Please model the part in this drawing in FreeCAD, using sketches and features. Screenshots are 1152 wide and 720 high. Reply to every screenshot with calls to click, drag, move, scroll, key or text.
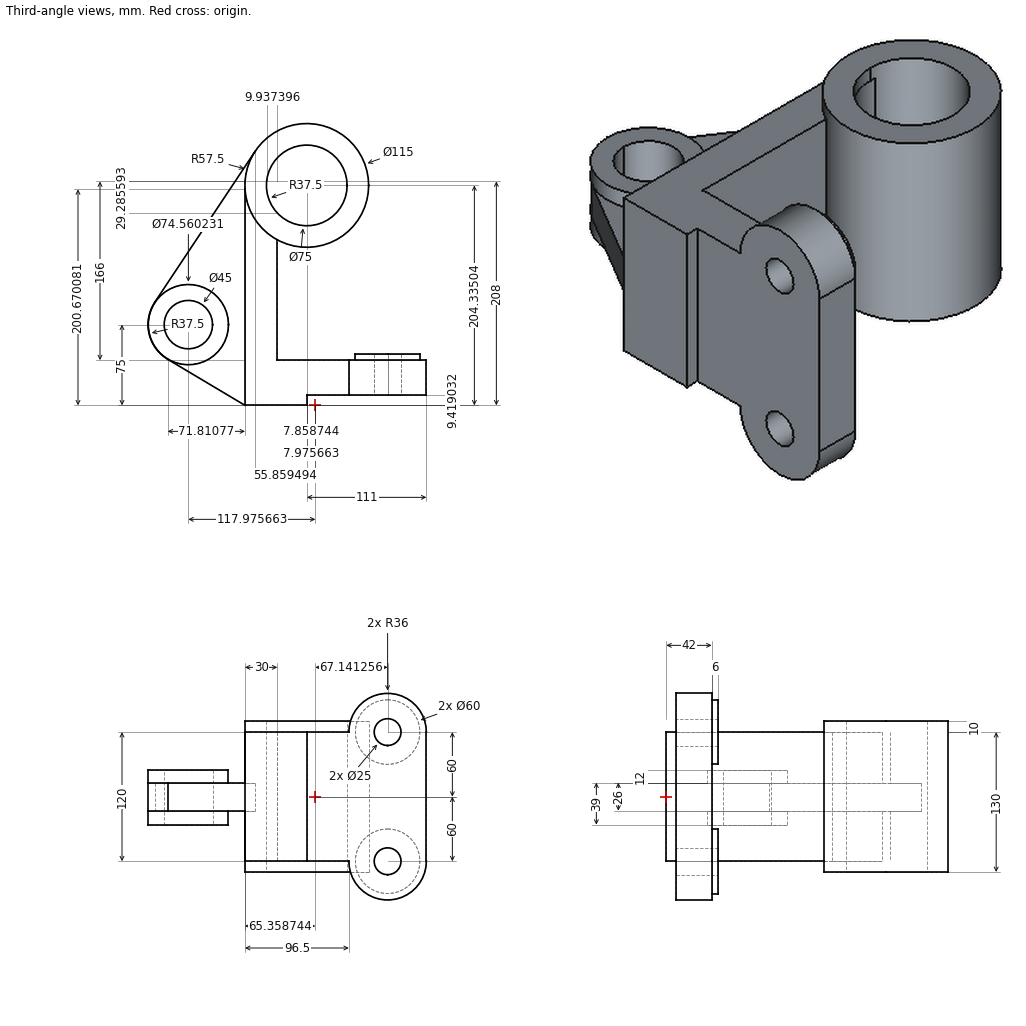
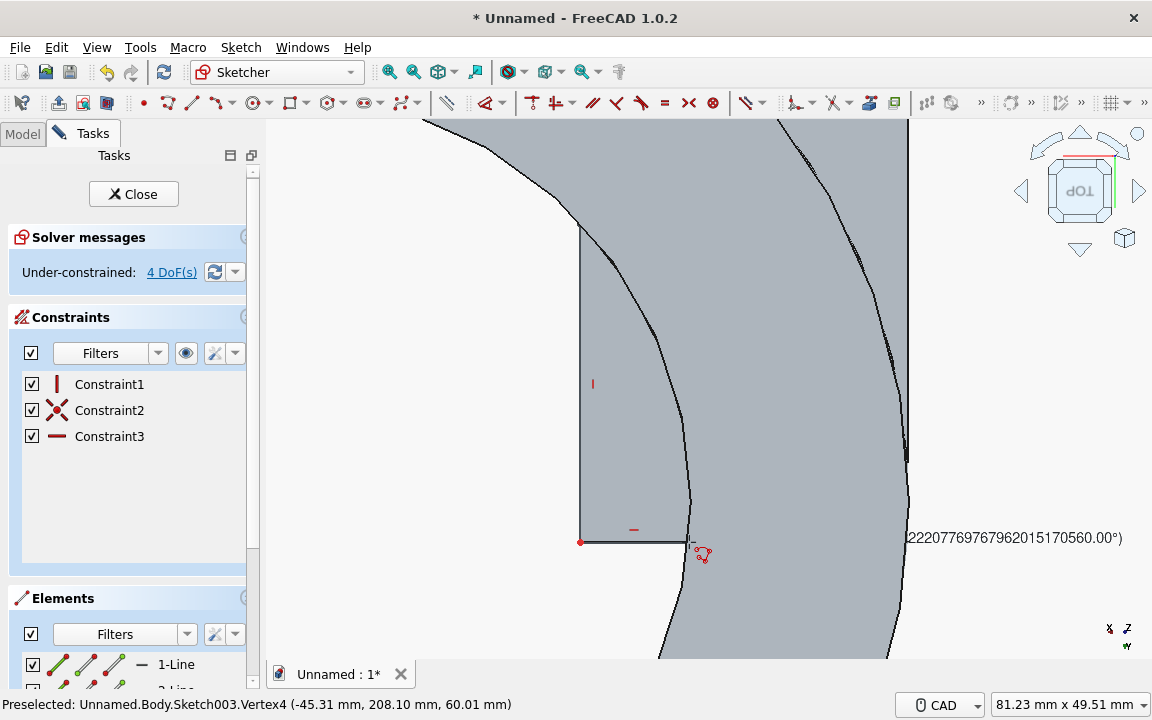
click(216, 104)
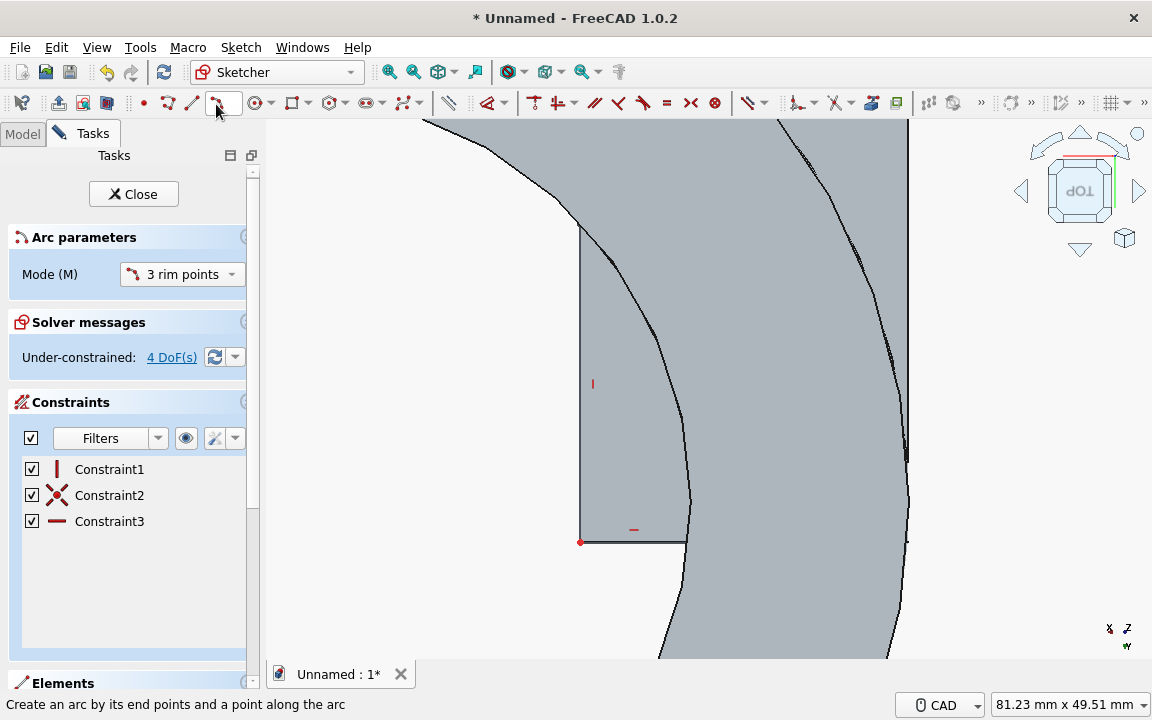
click(689, 543)
click(580, 224)
click(669, 371)
key(Escape)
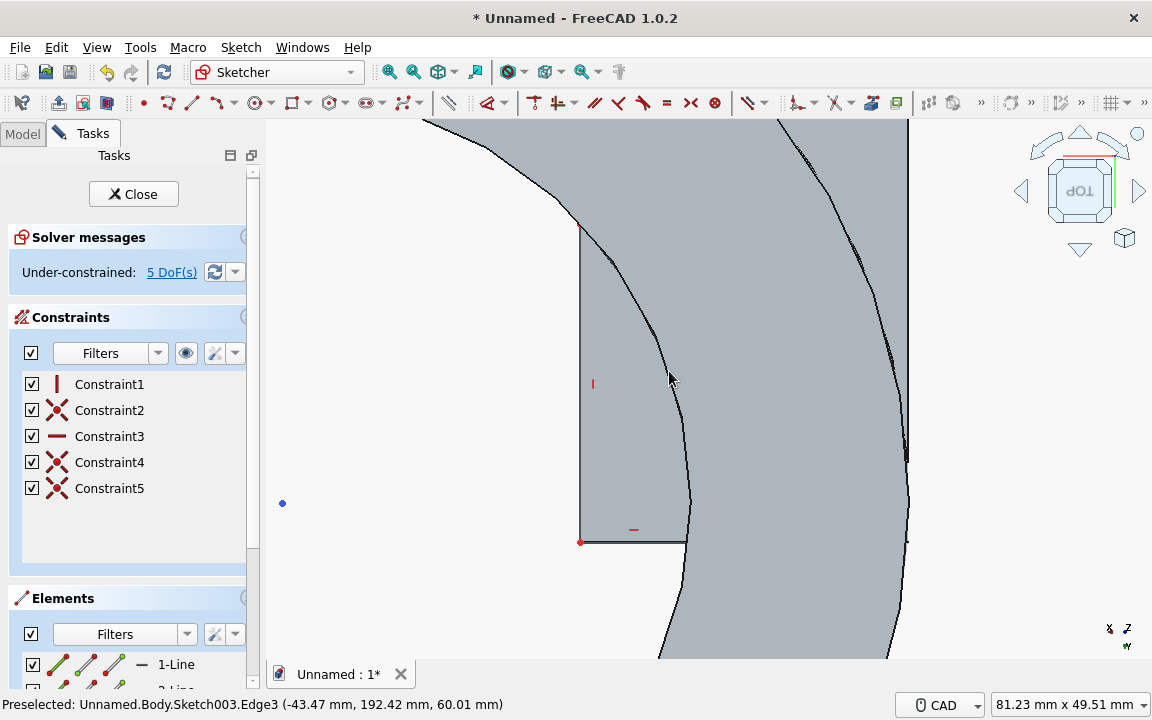
click(488, 104)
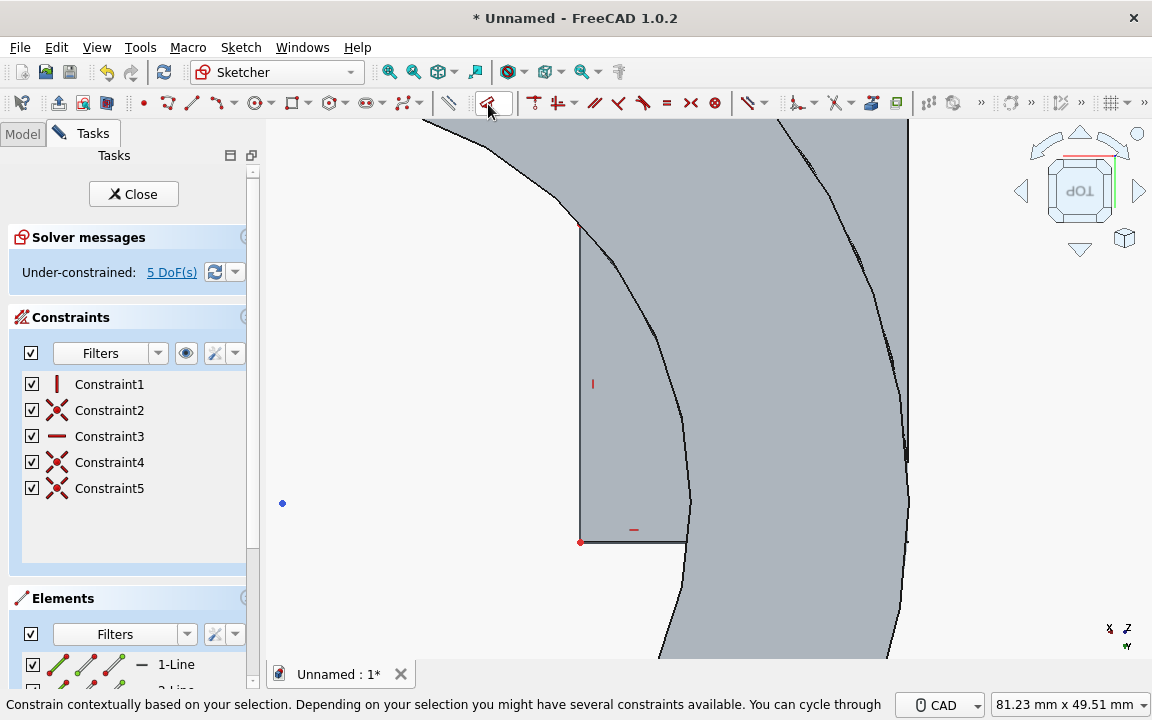
click(686, 439)
click(718, 434)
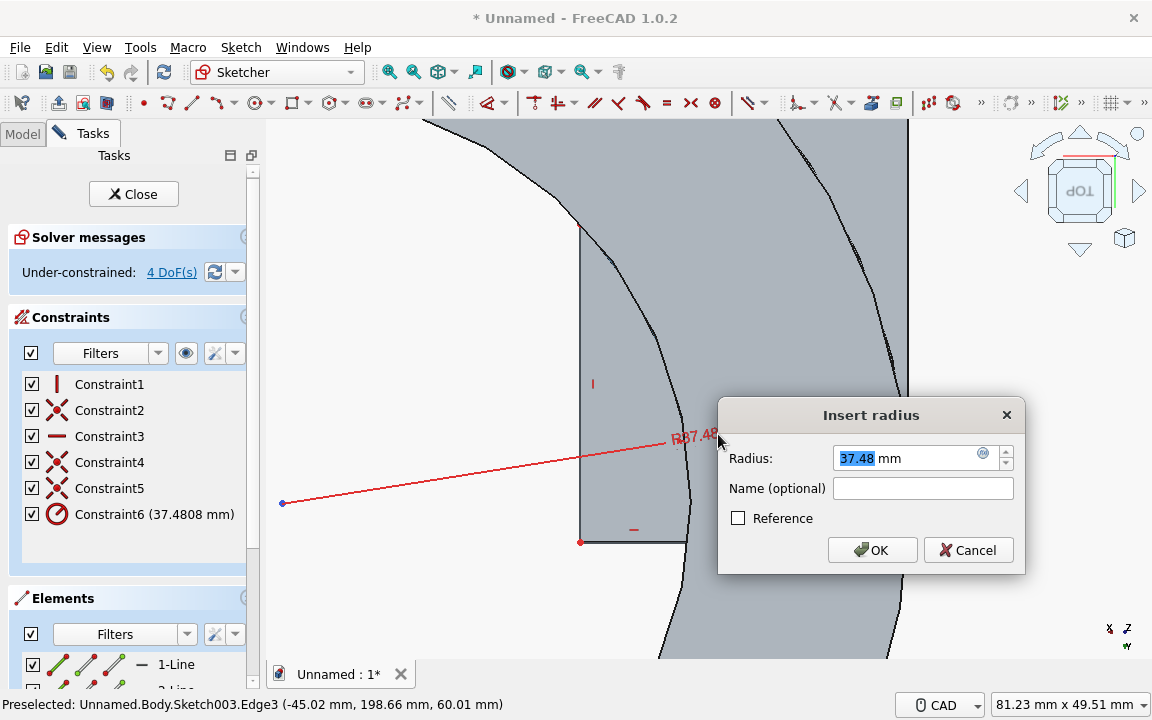
text(37.5)
key(Return)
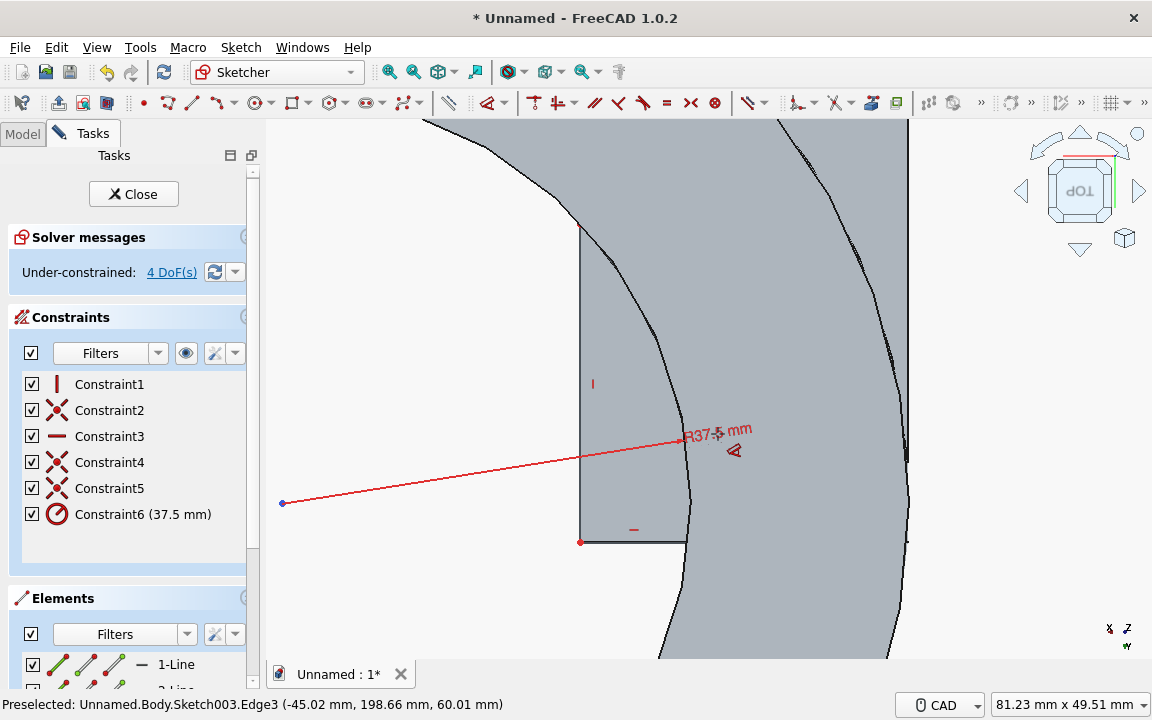
click(580, 543)
click(614, 345)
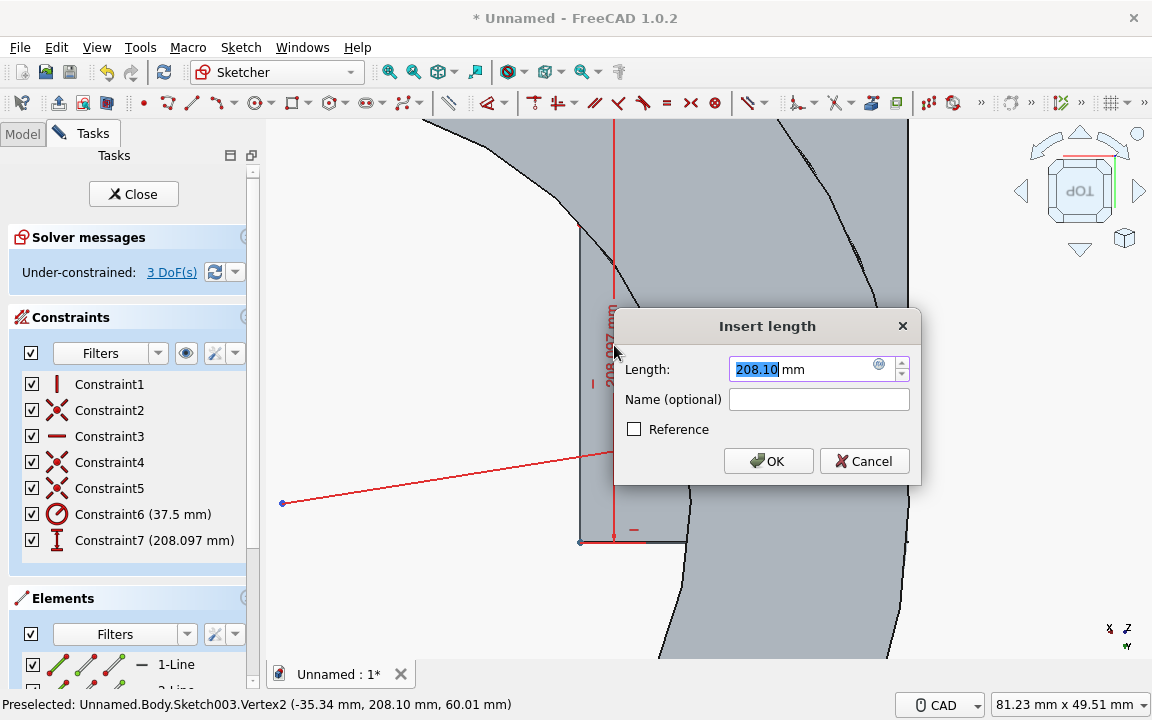
text(208)
key(Return)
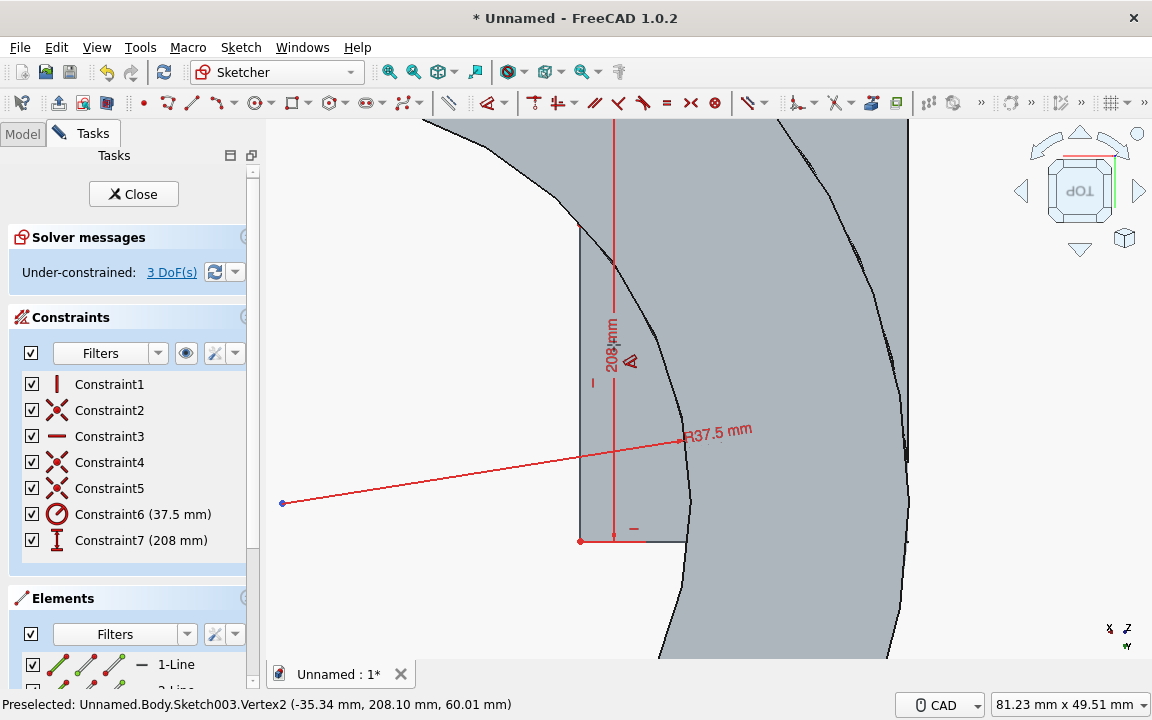
click(613, 542)
click(635, 576)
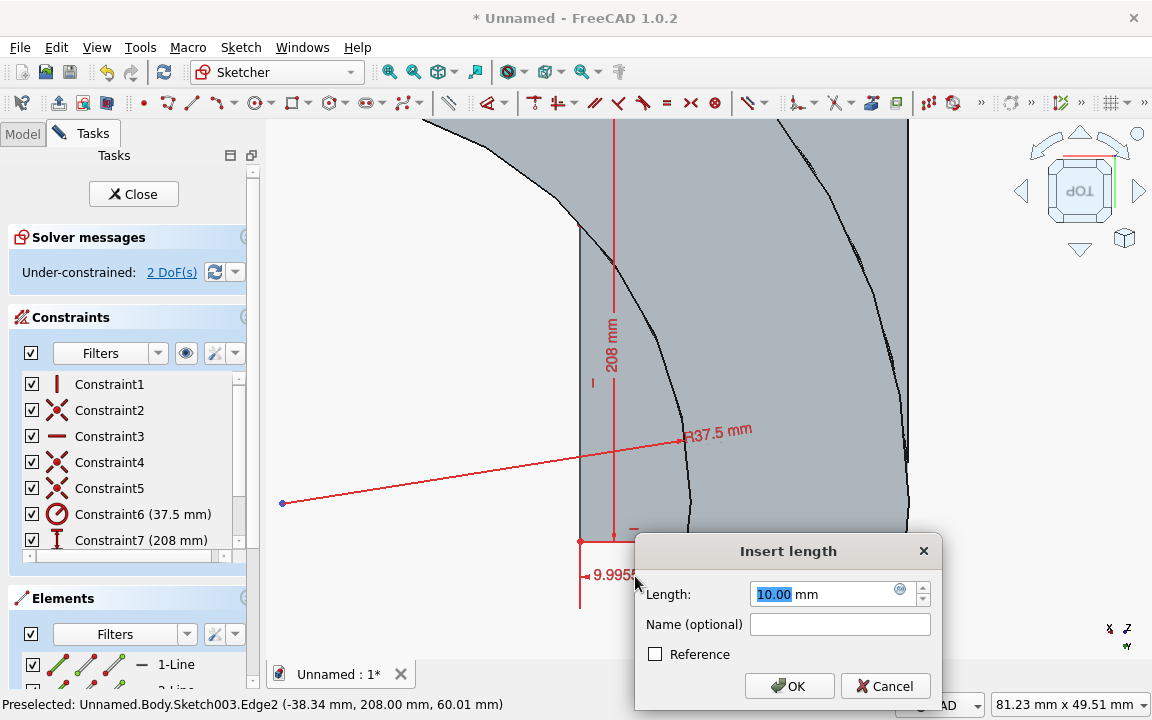
text(9.937396)
key(Return)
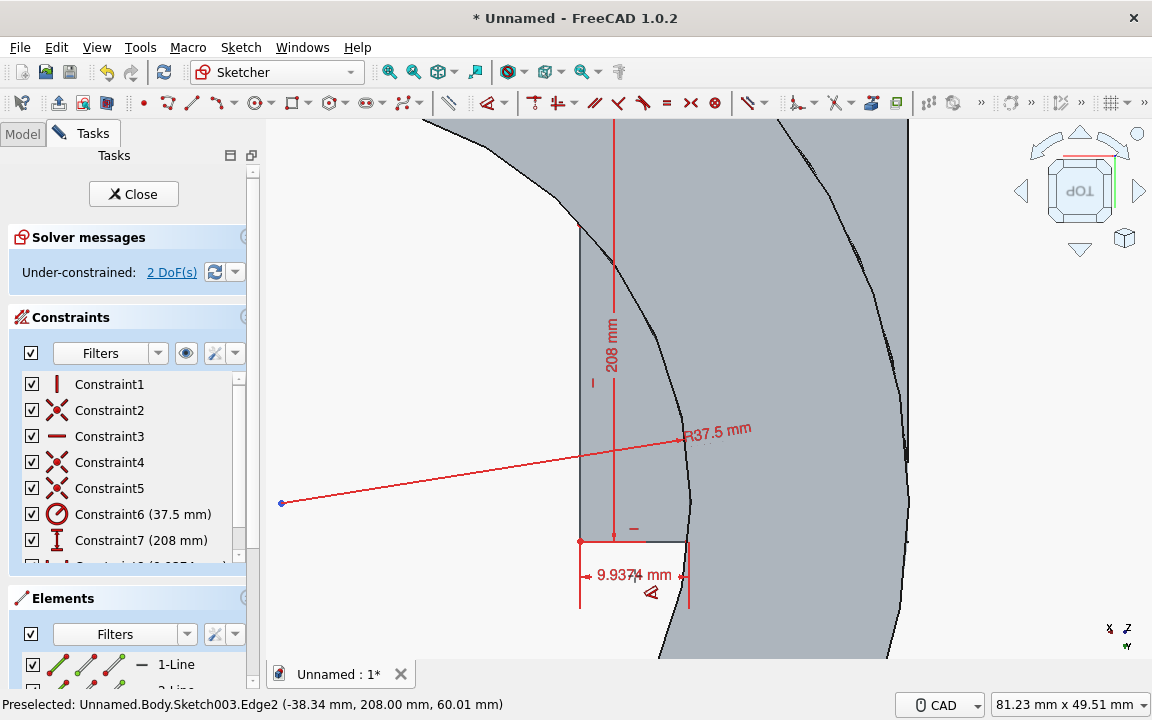
click(580, 319)
click(546, 383)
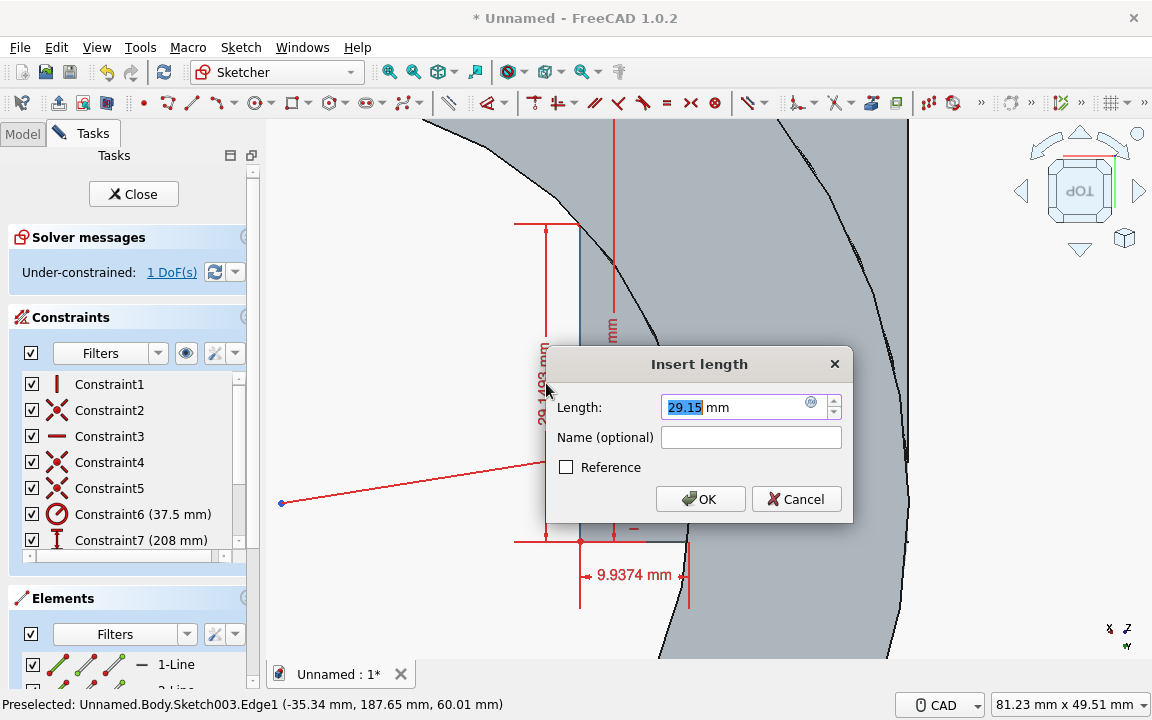
text(29.285593)
key(Return)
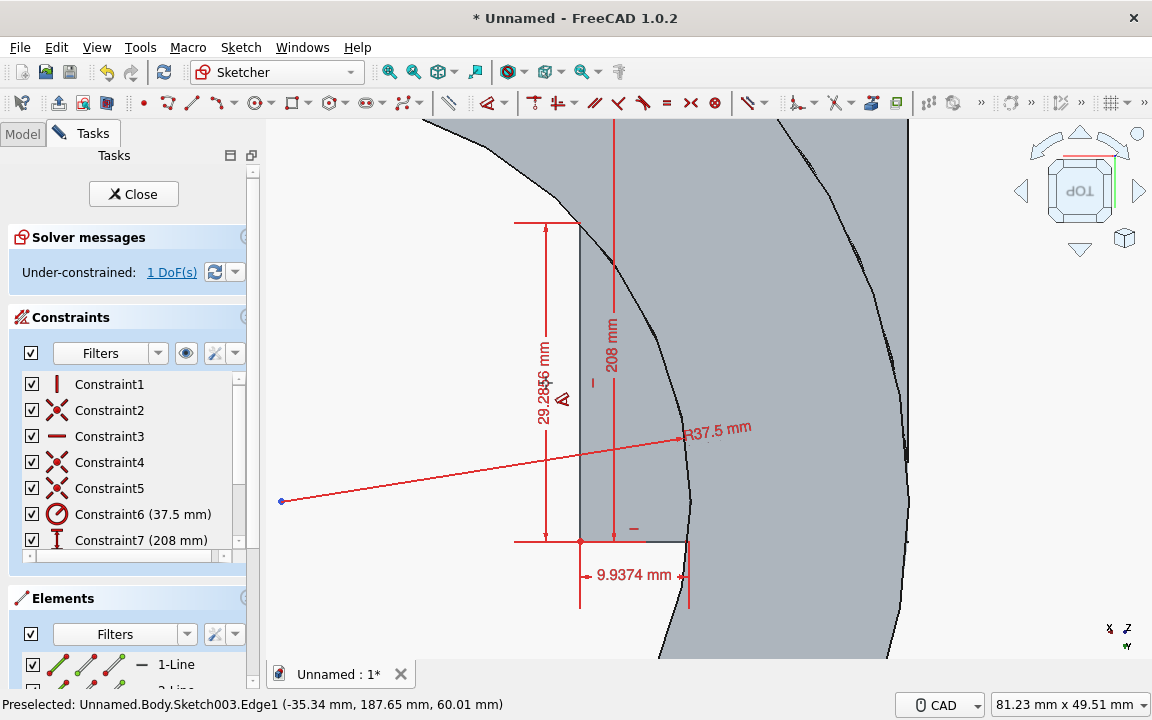
scroll(987, 420, down, 1)